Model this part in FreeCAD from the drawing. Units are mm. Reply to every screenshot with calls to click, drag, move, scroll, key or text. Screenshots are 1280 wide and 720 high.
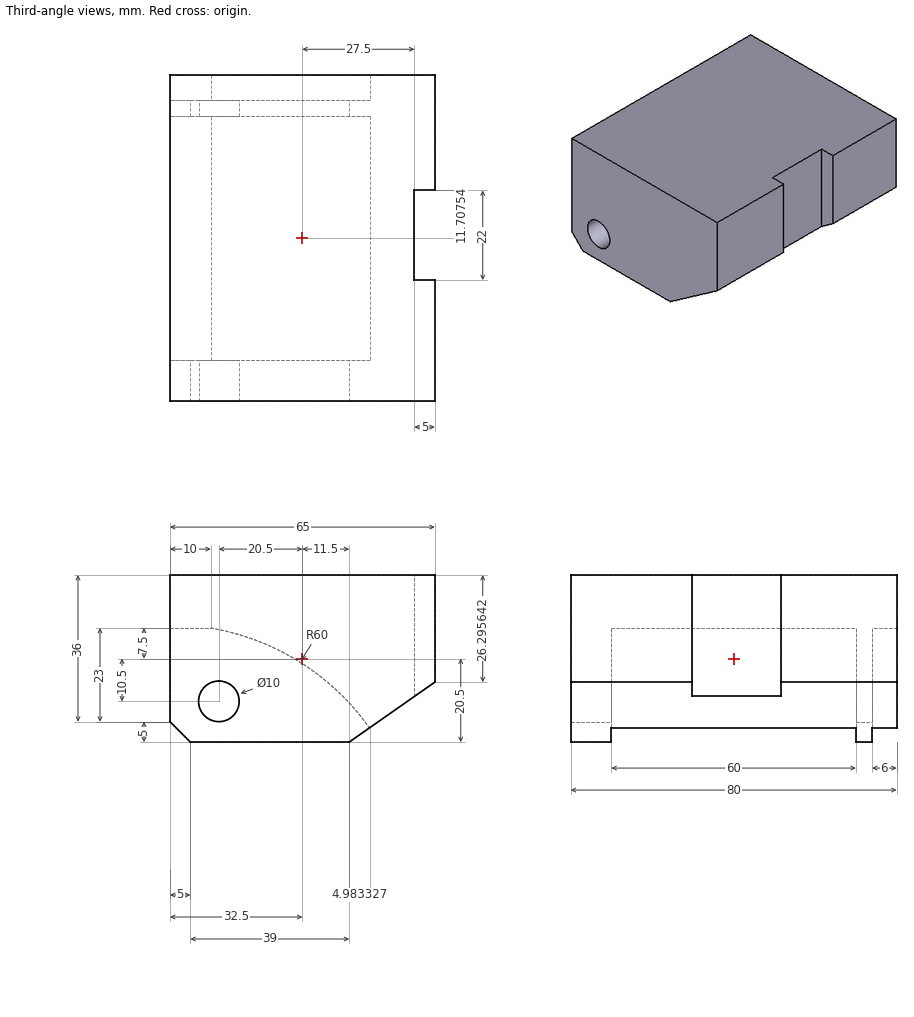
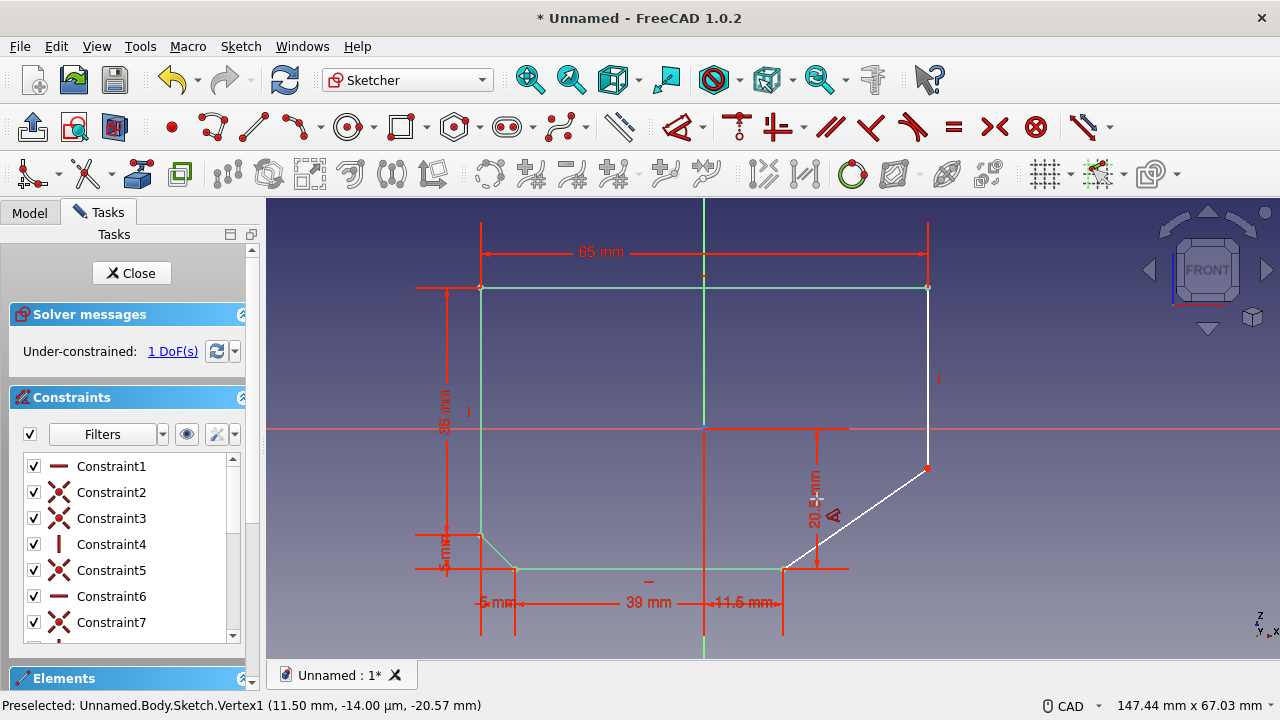
click(928, 342)
click(962, 378)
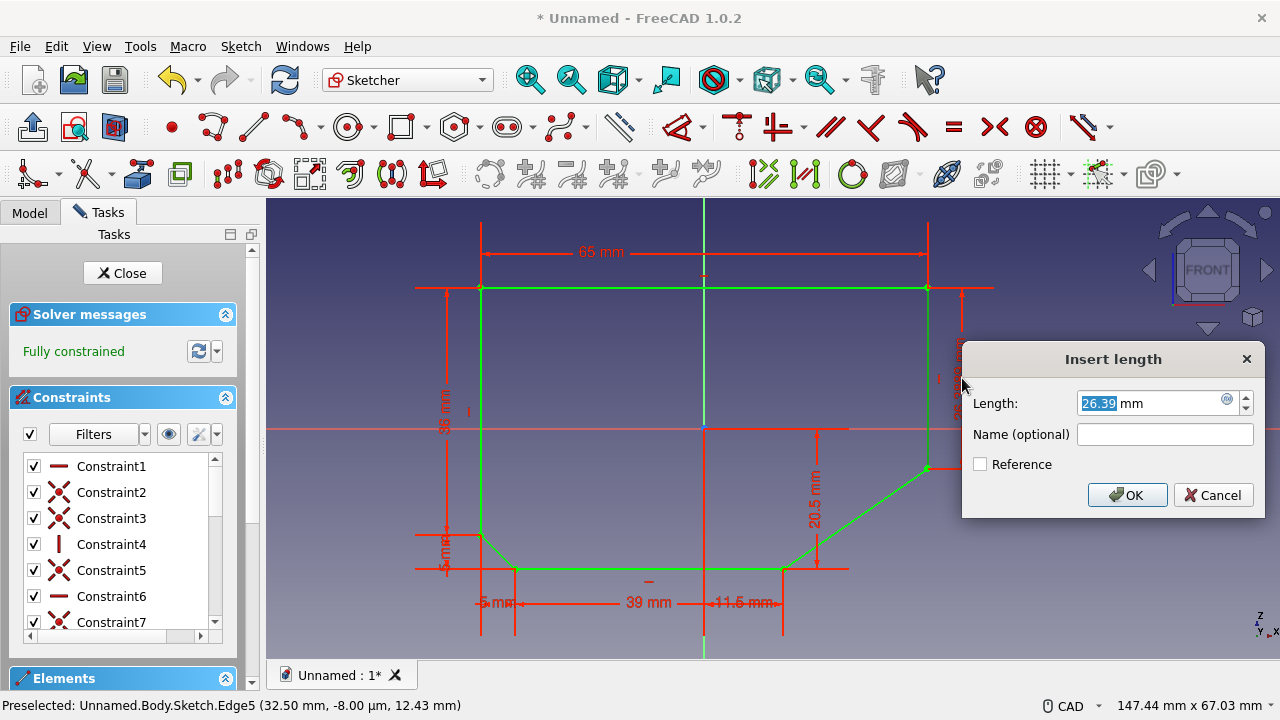
text(26.295642)
key(Return)
key(Escape)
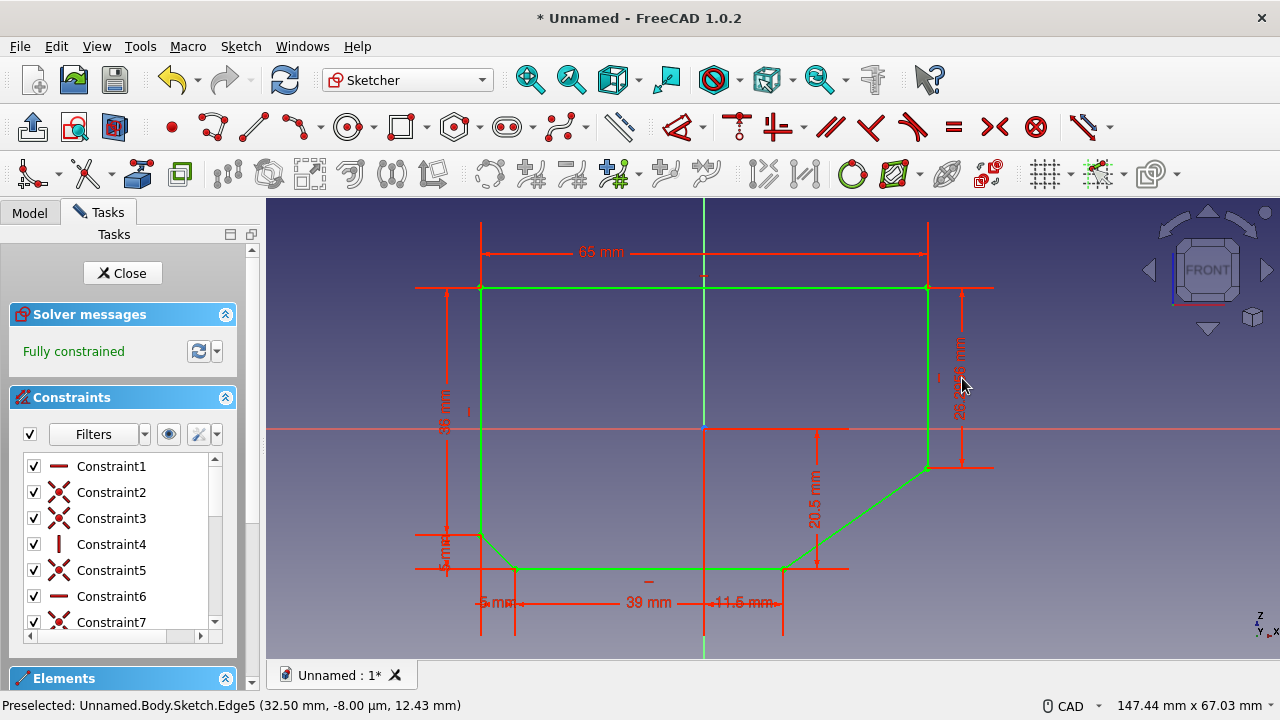
click(123, 273)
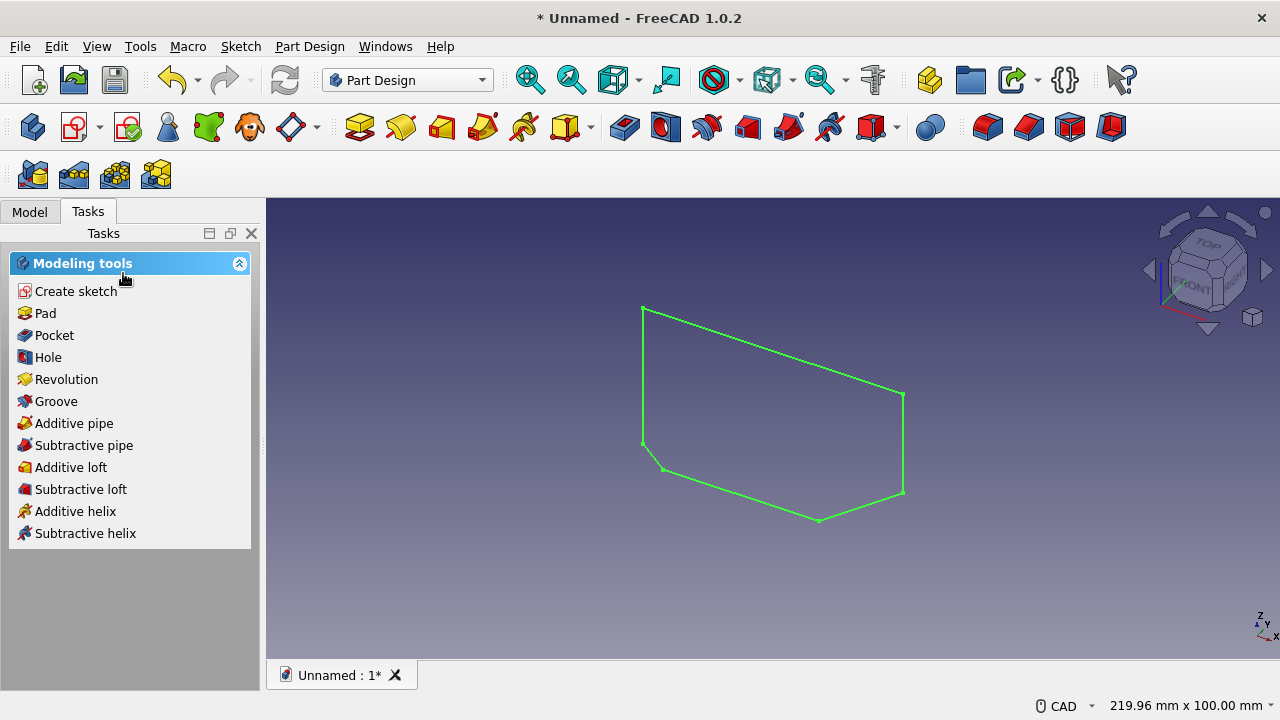
click(360, 128)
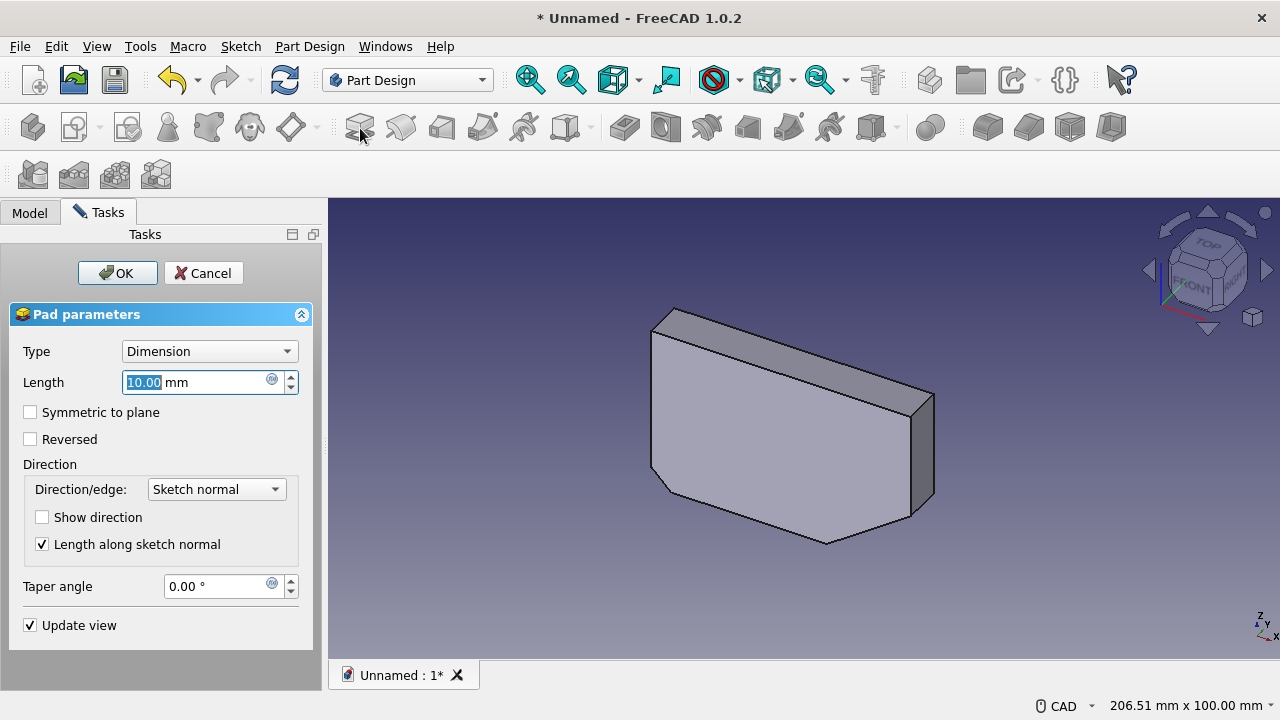
text(80)
key(Tab)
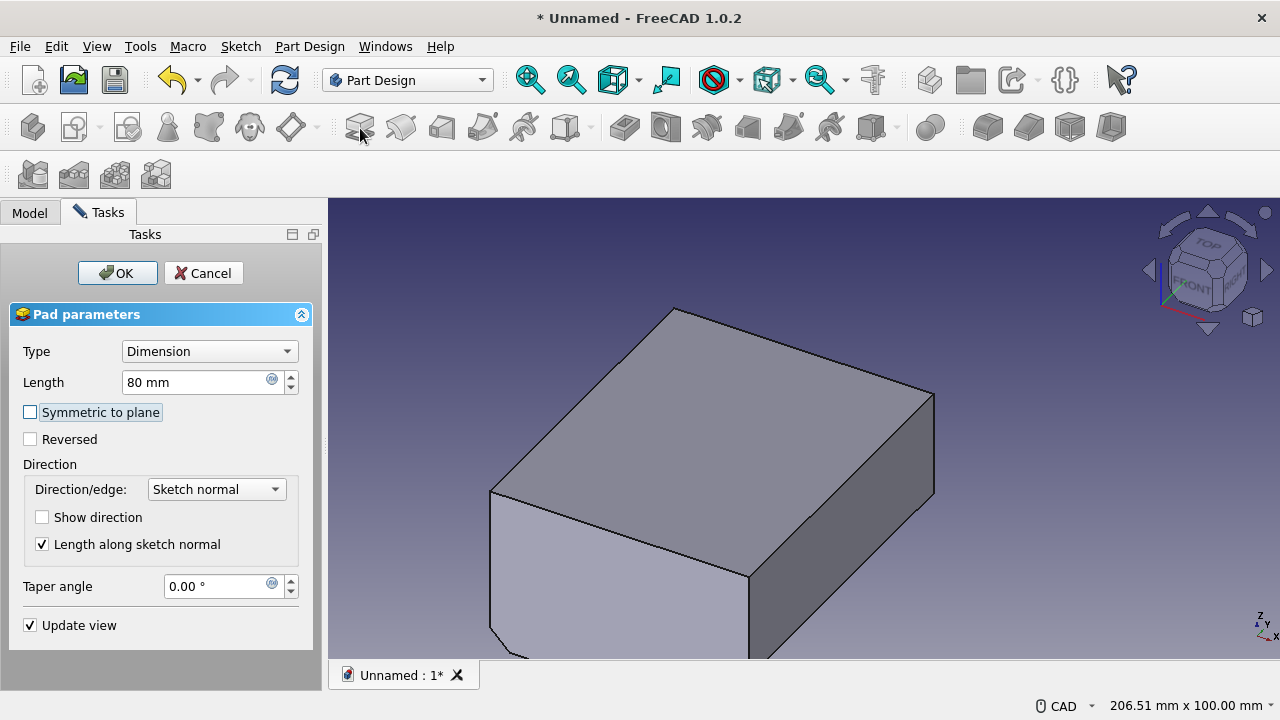
click(31, 412)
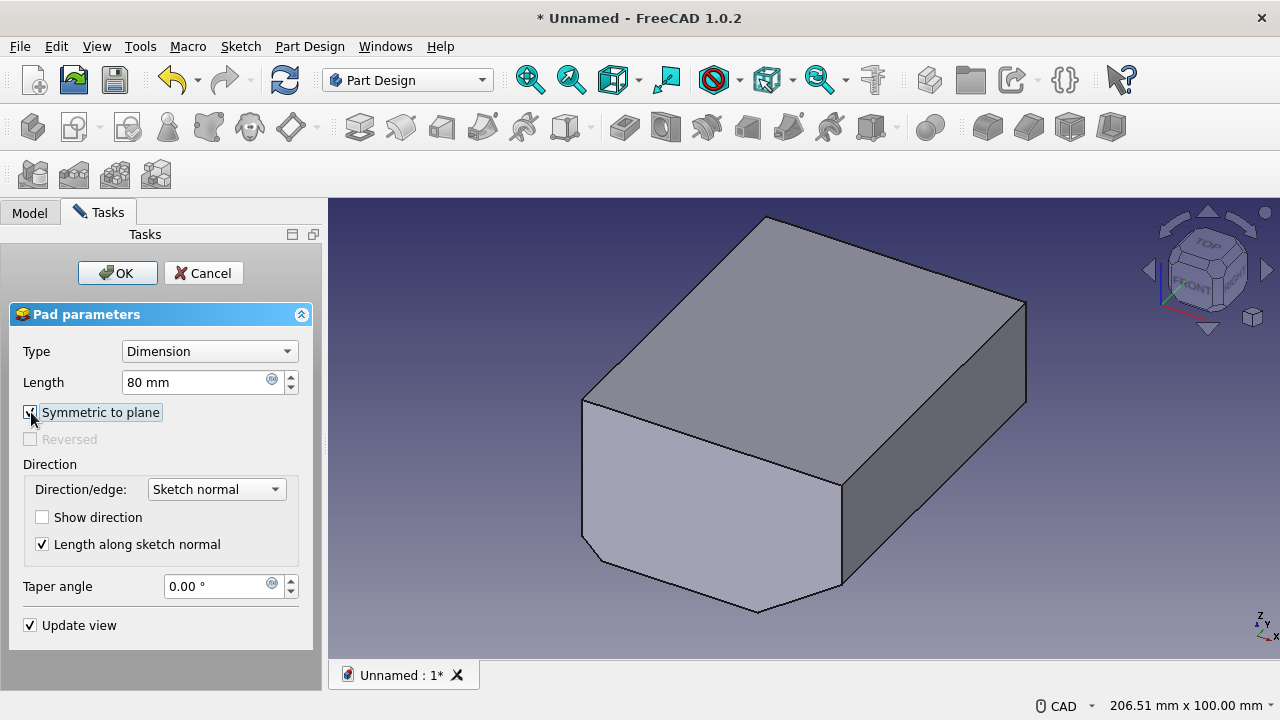
click(118, 273)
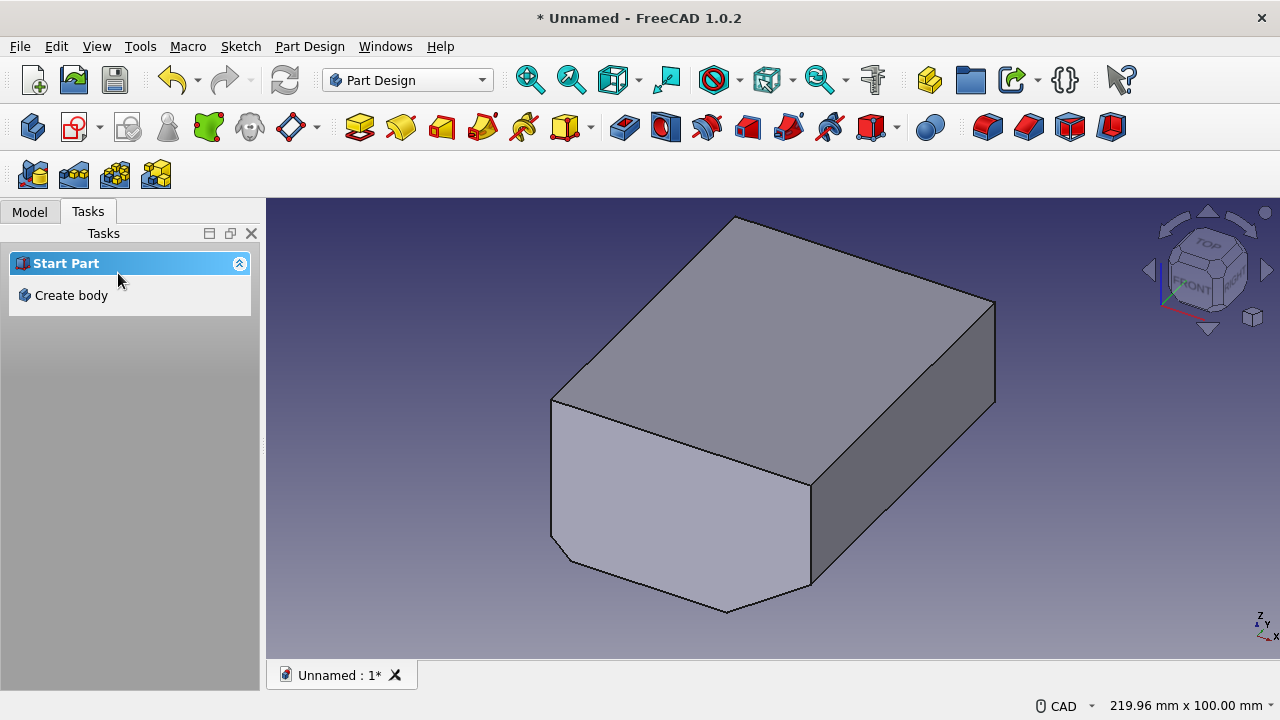
click(74, 128)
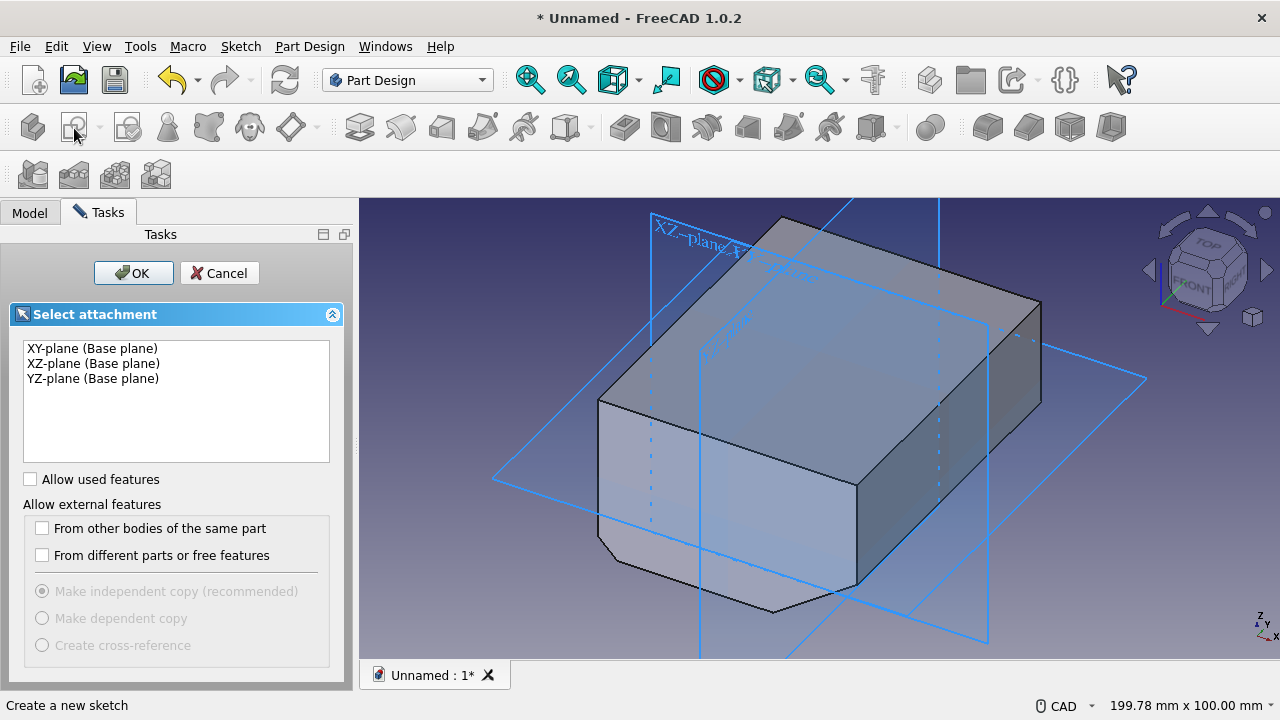
click(84, 348)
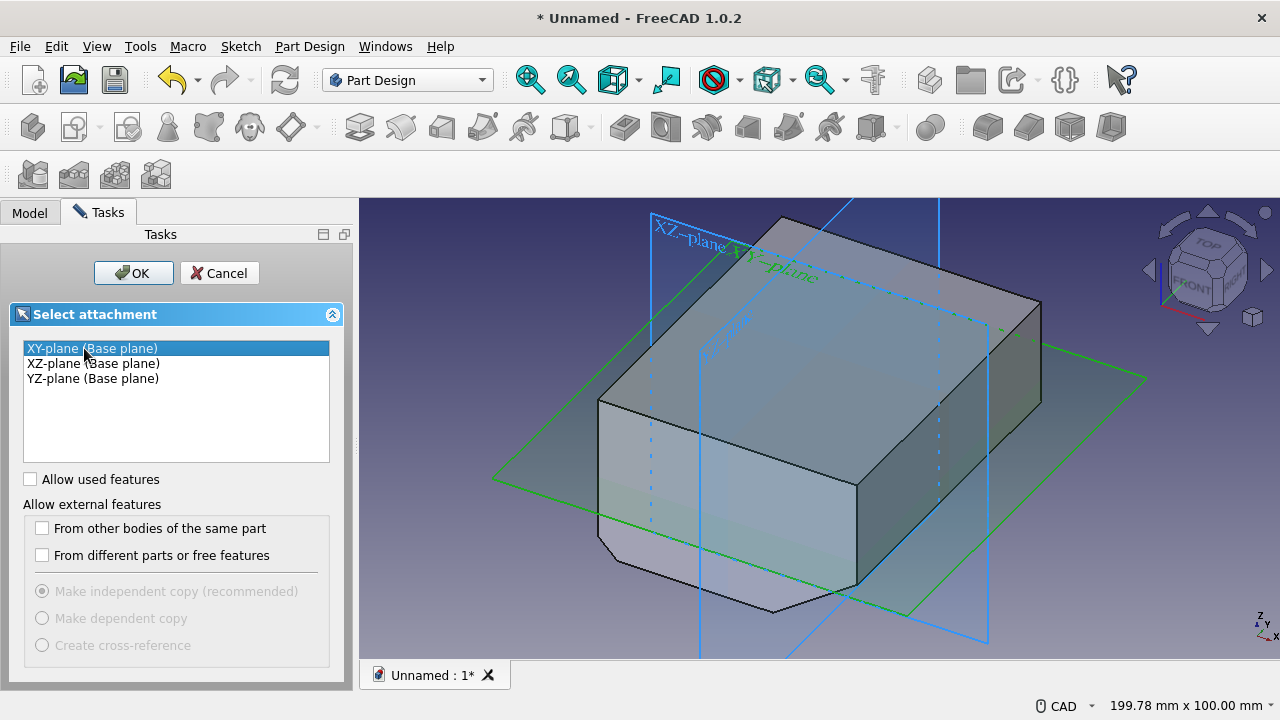
click(134, 273)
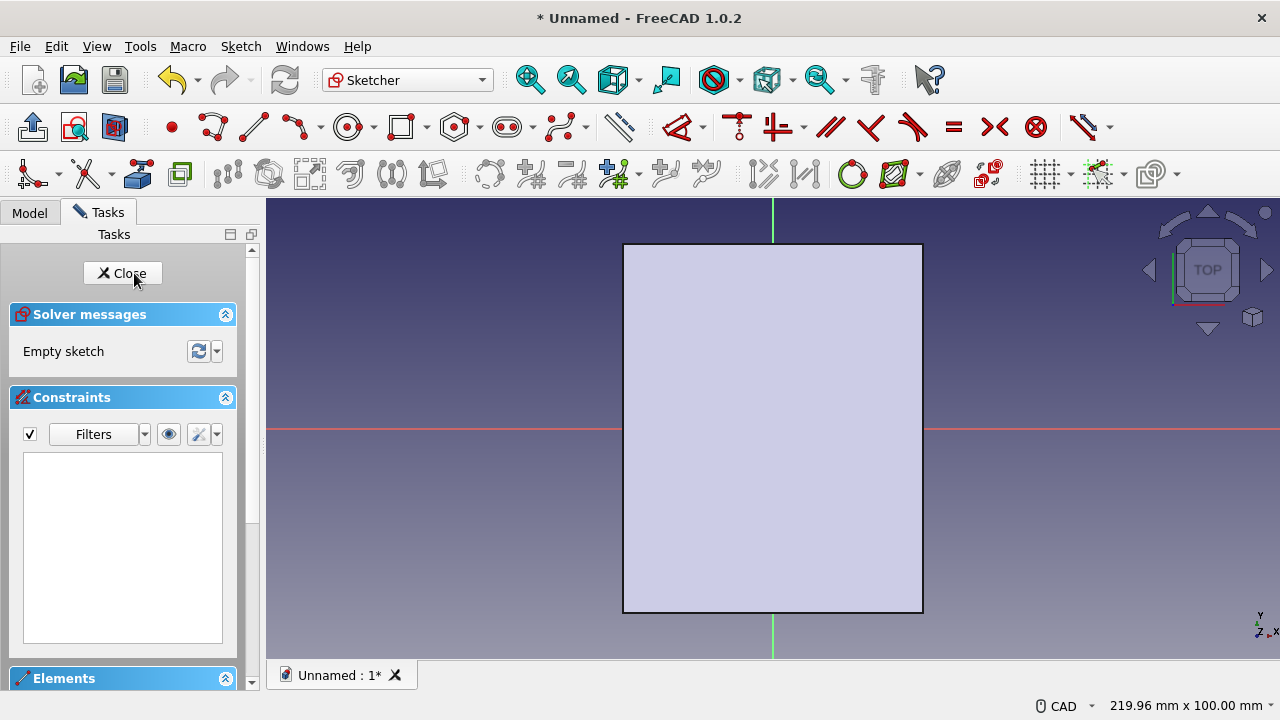
key(q)
key(s)